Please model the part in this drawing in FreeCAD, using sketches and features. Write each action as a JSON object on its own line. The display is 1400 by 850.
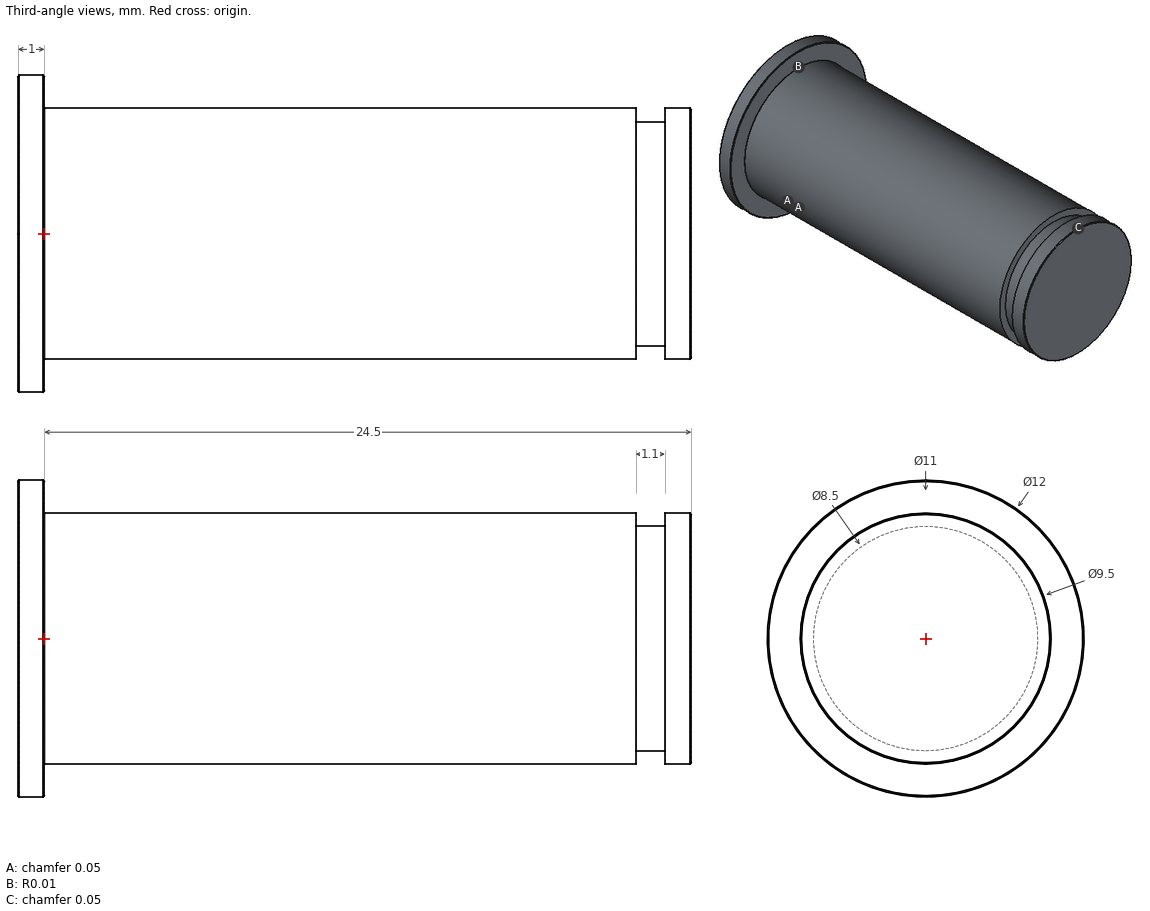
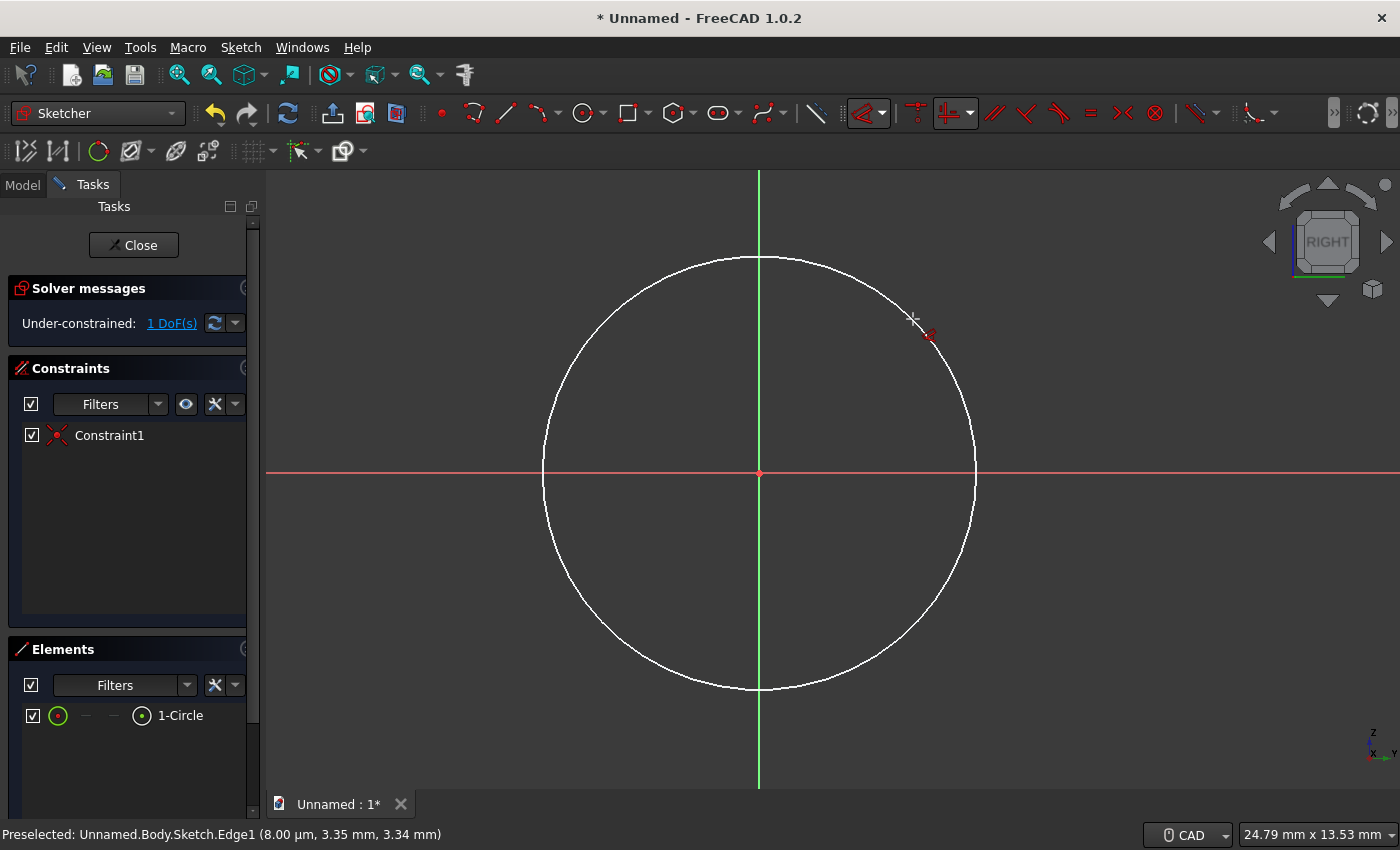
{"action": "left_click", "coordinate": [912, 319]}
{"action": "left_click", "coordinate": [935, 296]}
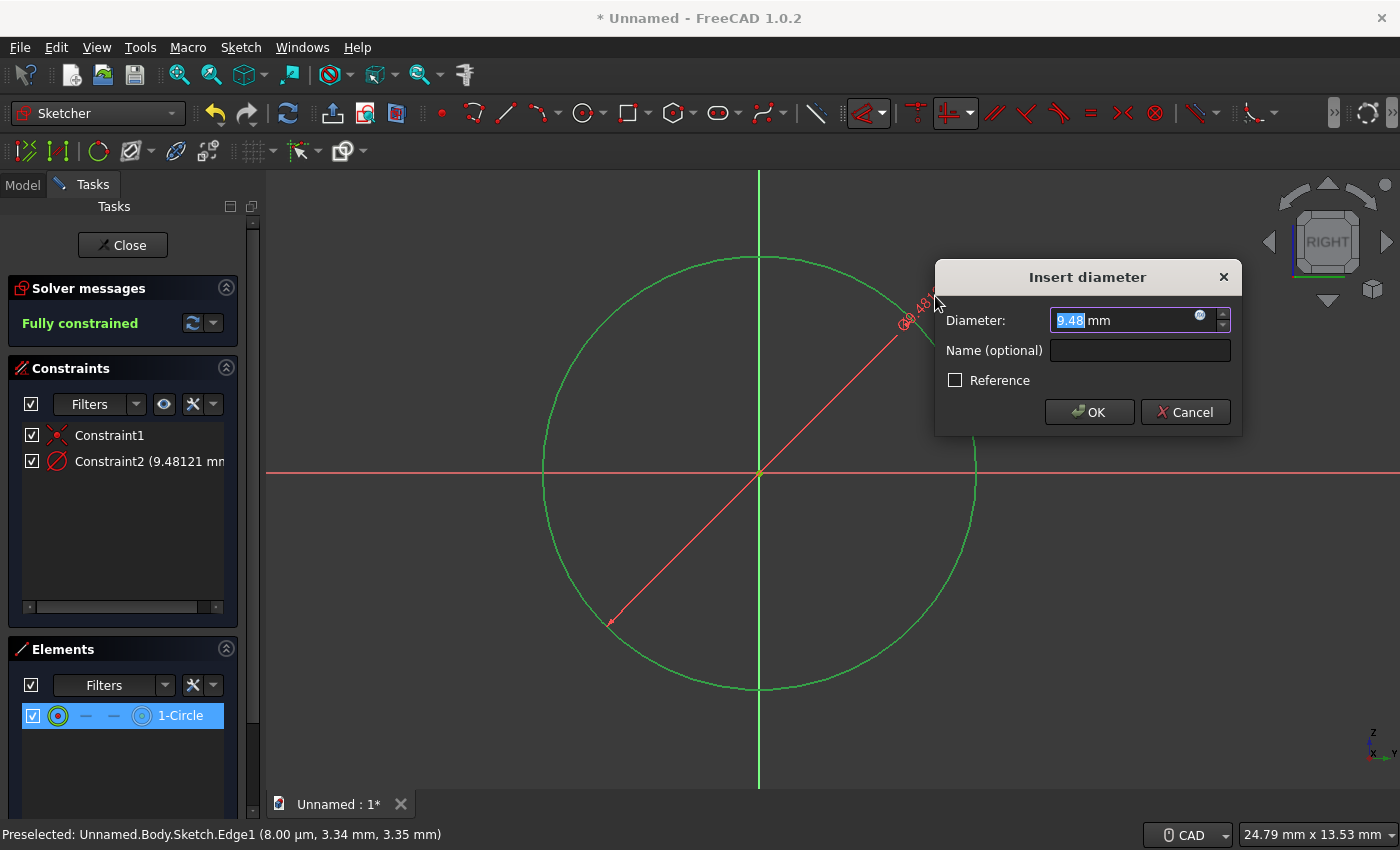
{"action": "type", "text": "9.5"}
{"action": "key", "text": "Return"}
{"action": "key", "text": "Escape"}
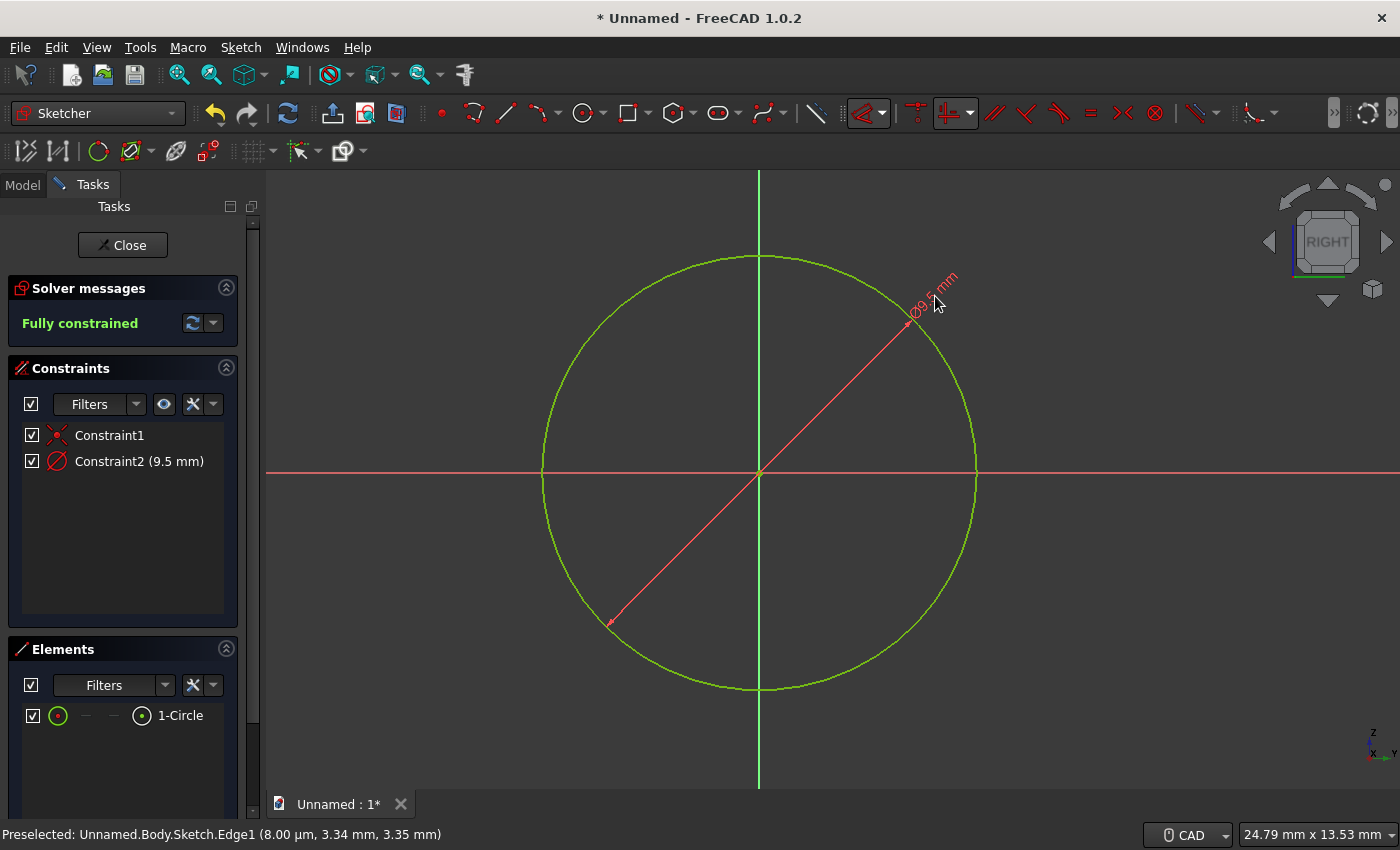
{"action": "left_click", "coordinate": [123, 245]}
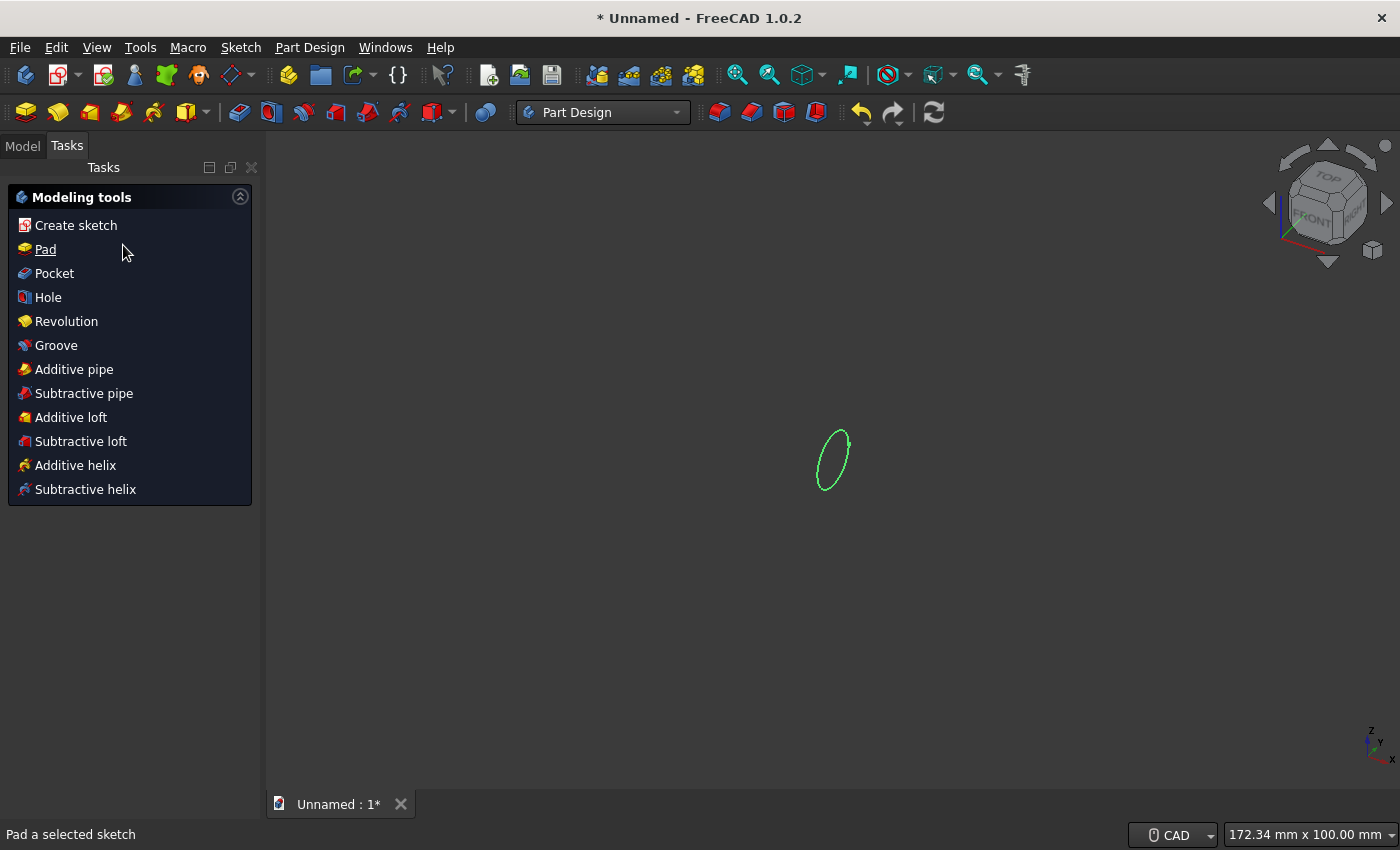
{"action": "left_click", "coordinate": [26, 112]}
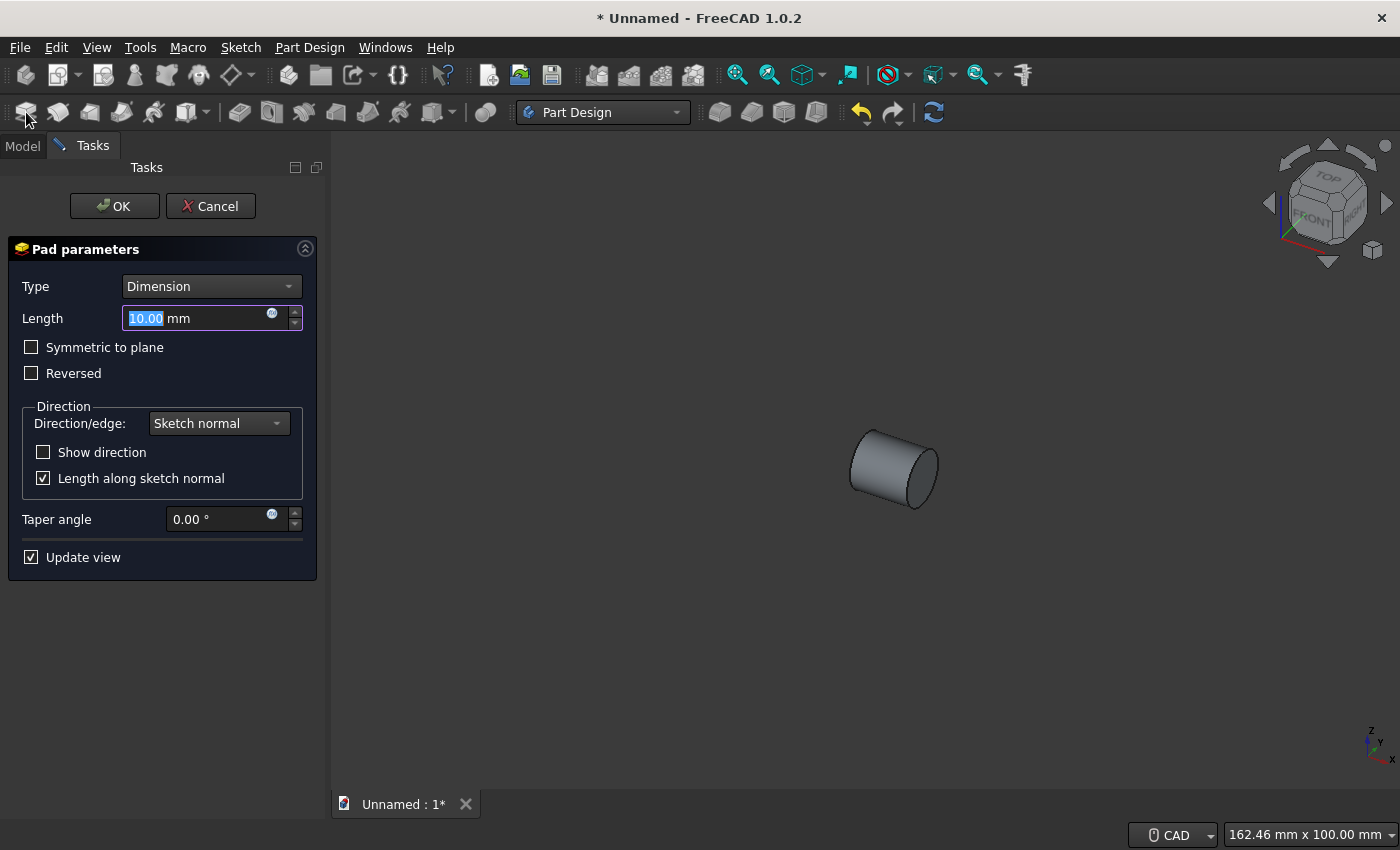
{"action": "type", "text": "24.5"}
{"action": "key", "text": "Tab"}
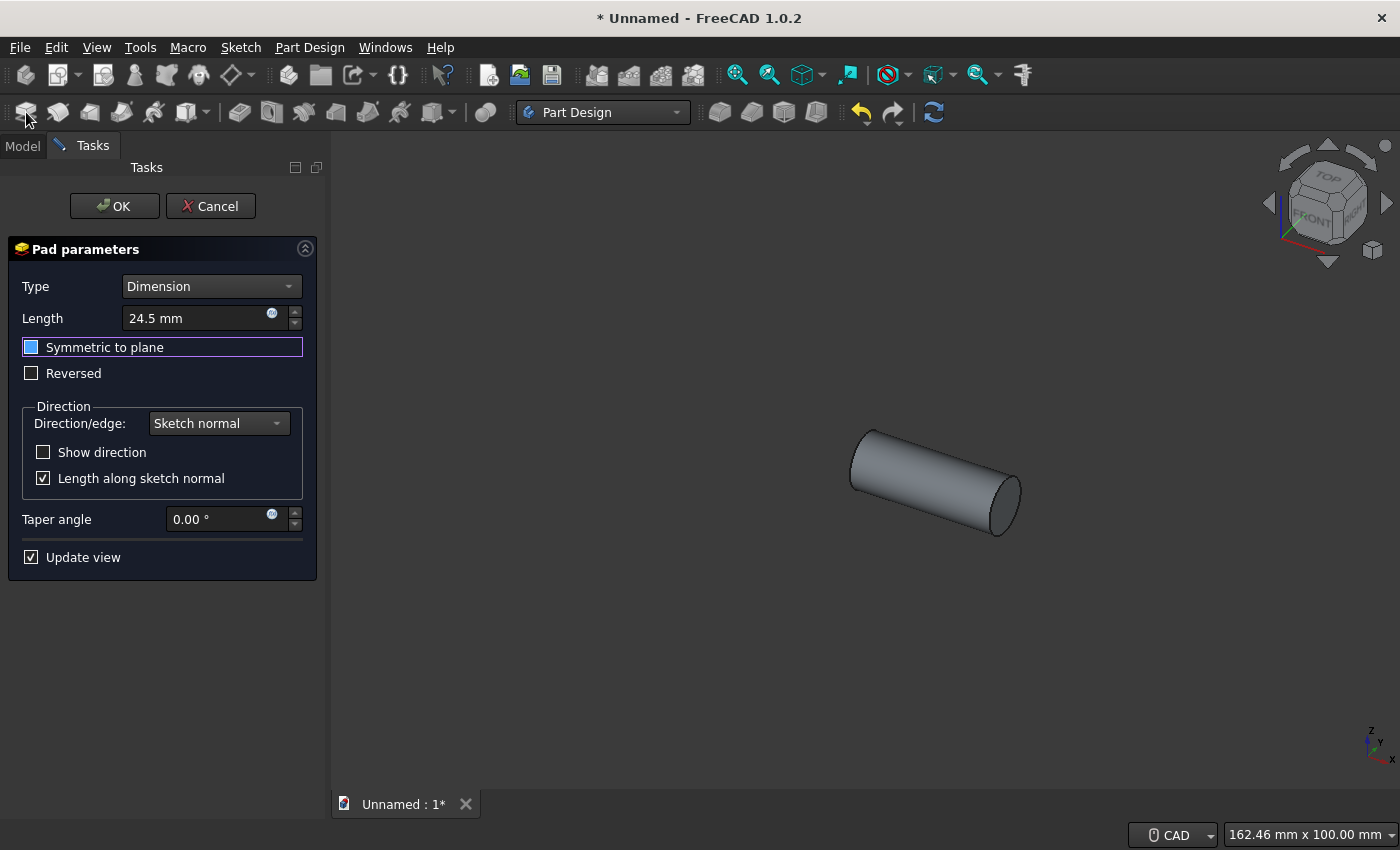
{"action": "left_click", "coordinate": [115, 206]}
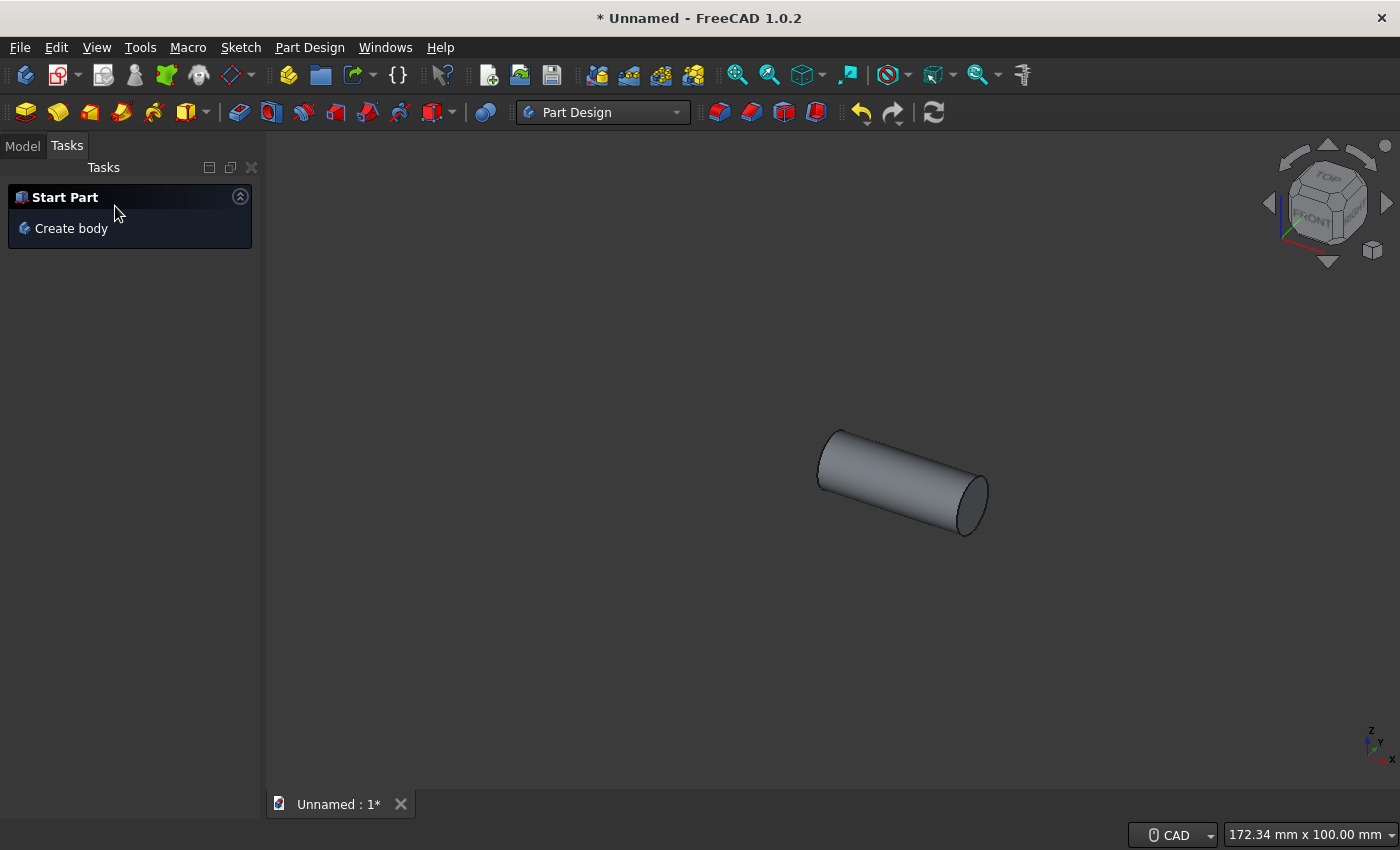
{"action": "left_click", "coordinate": [738, 76]}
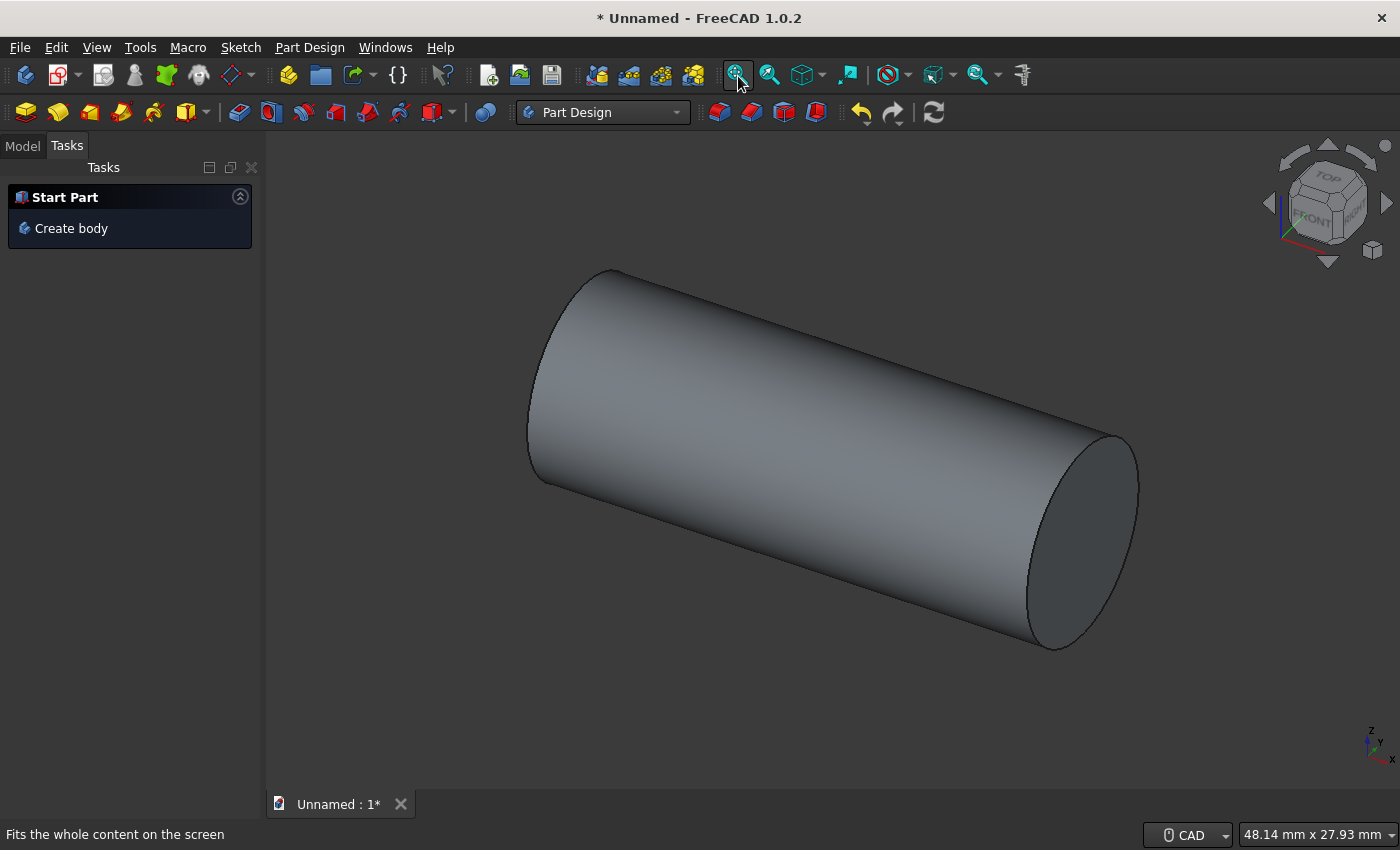
{"action": "key", "text": "6"}